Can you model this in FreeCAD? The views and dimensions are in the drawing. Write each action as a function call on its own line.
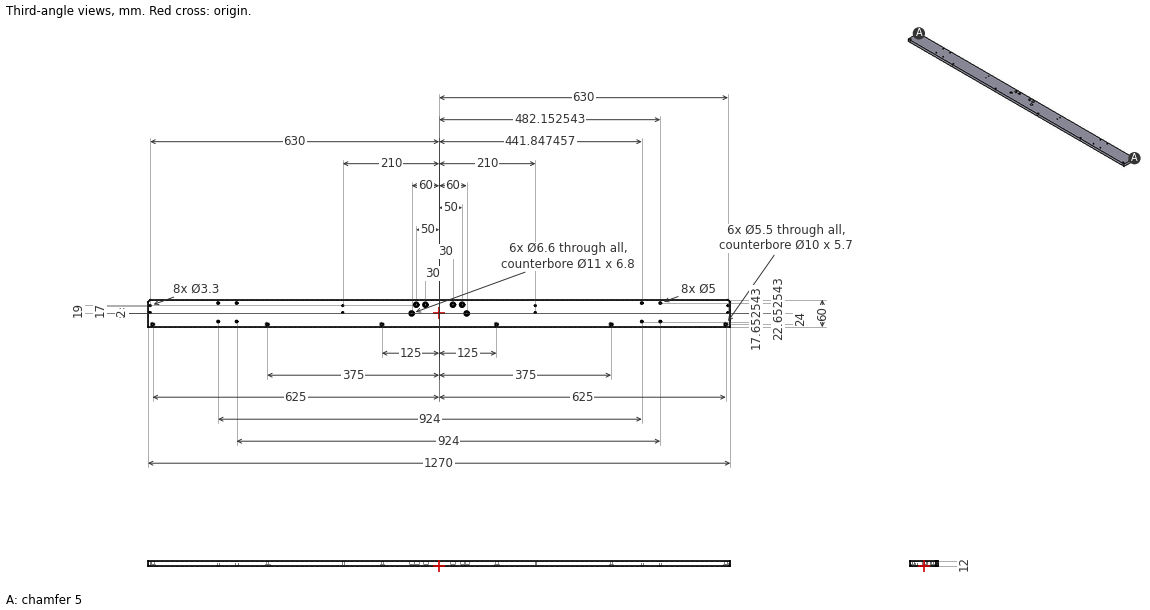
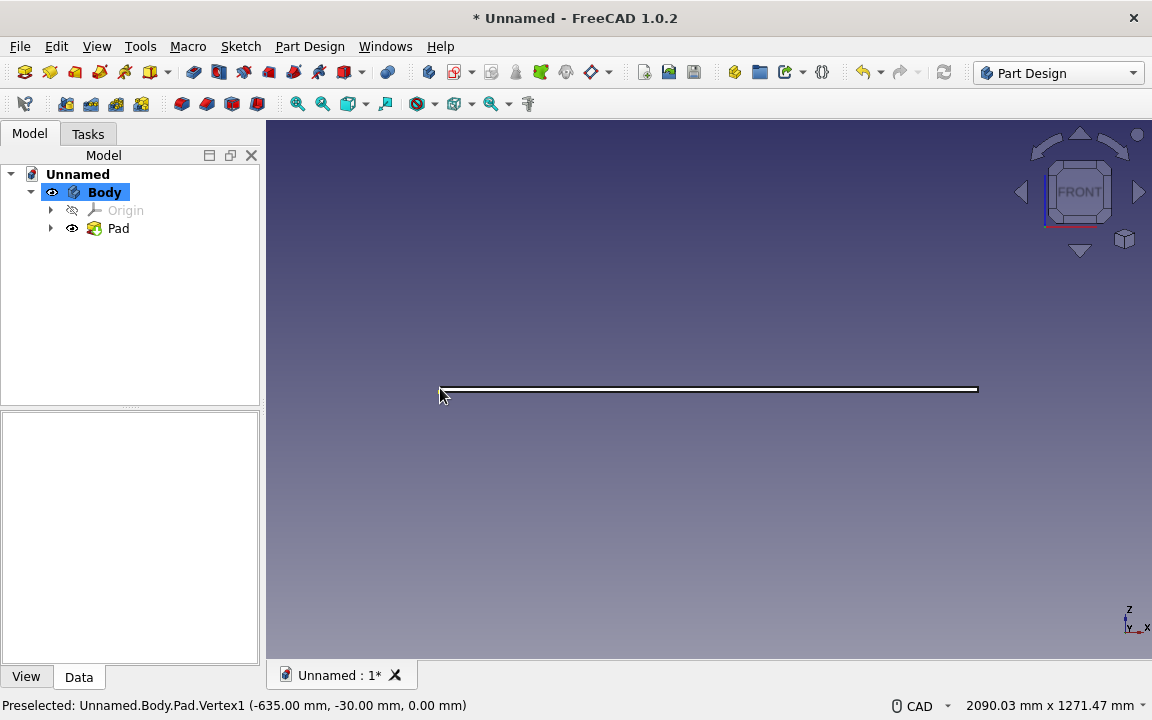
key(3)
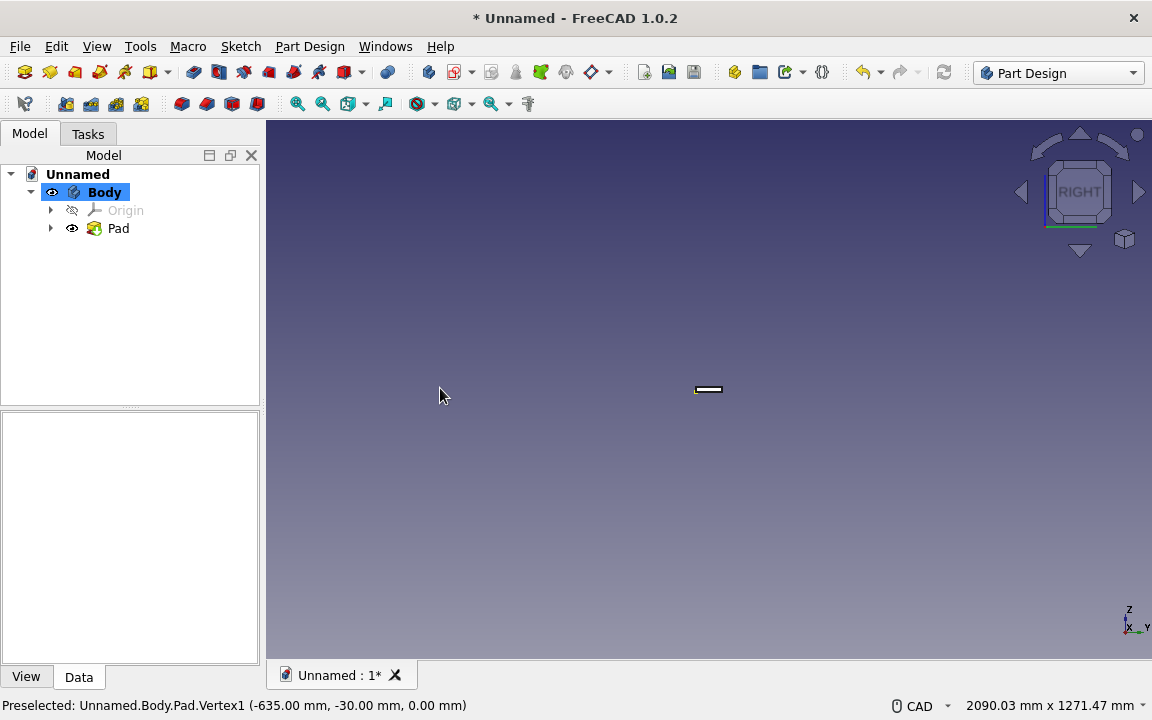
key(v)
key(f)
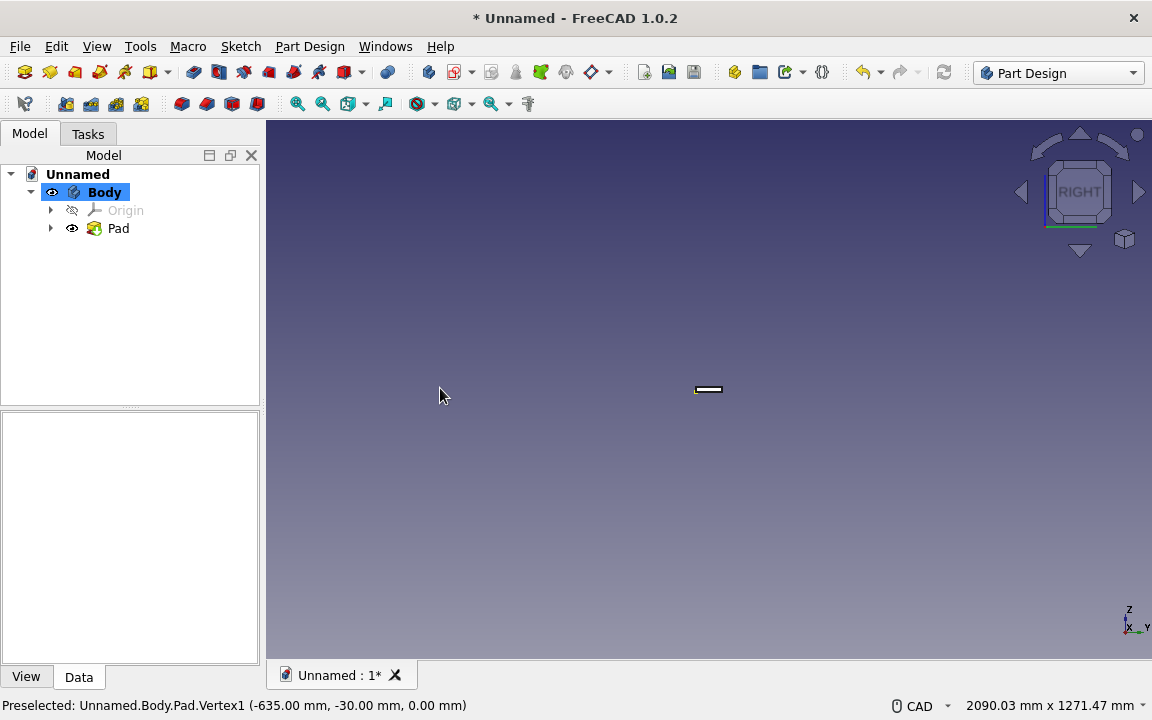
scroll(722, 388, up, 11)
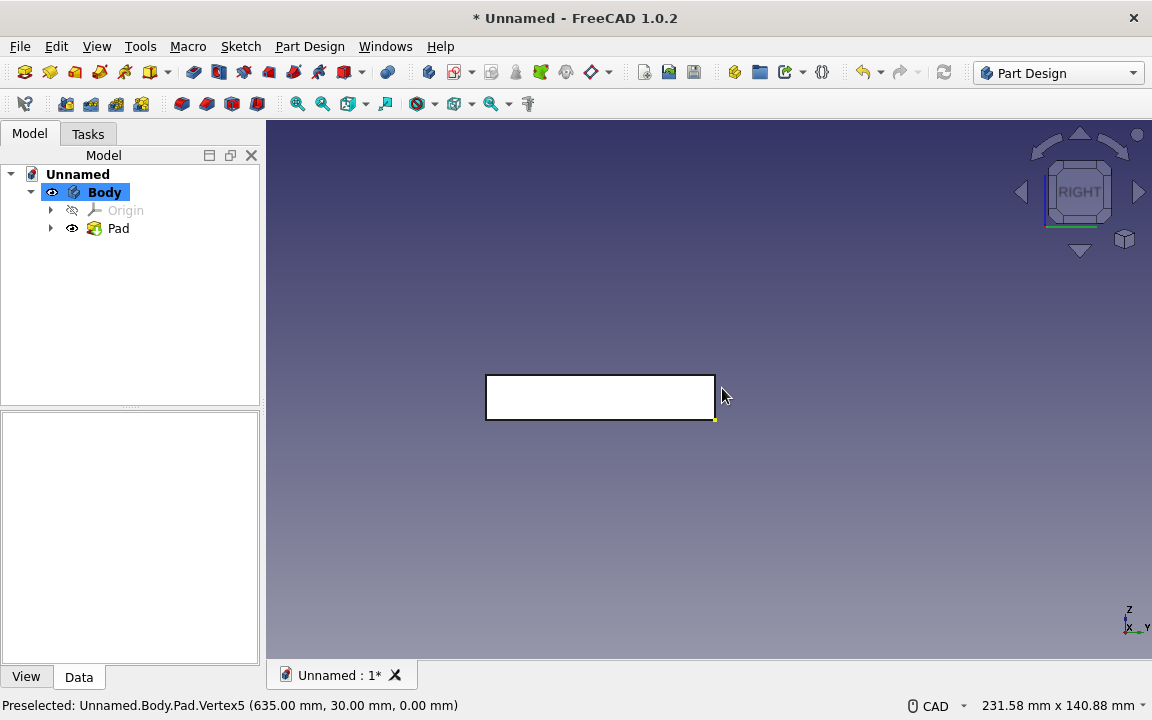
click(715, 397)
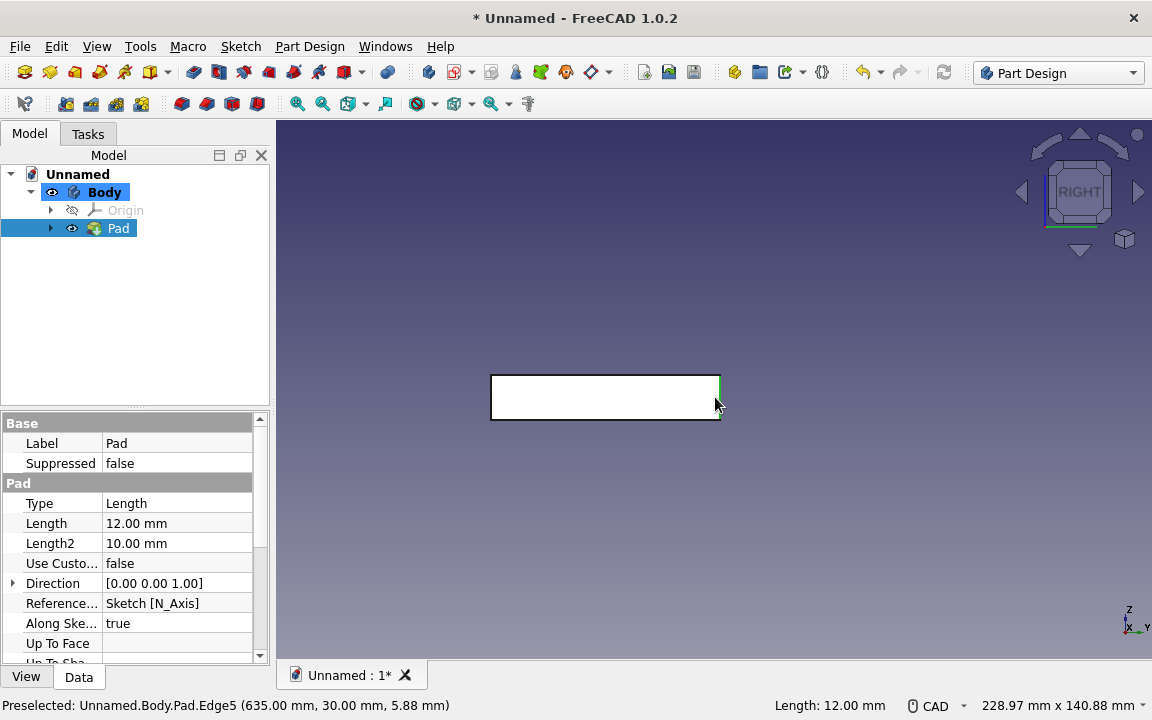
click(298, 104)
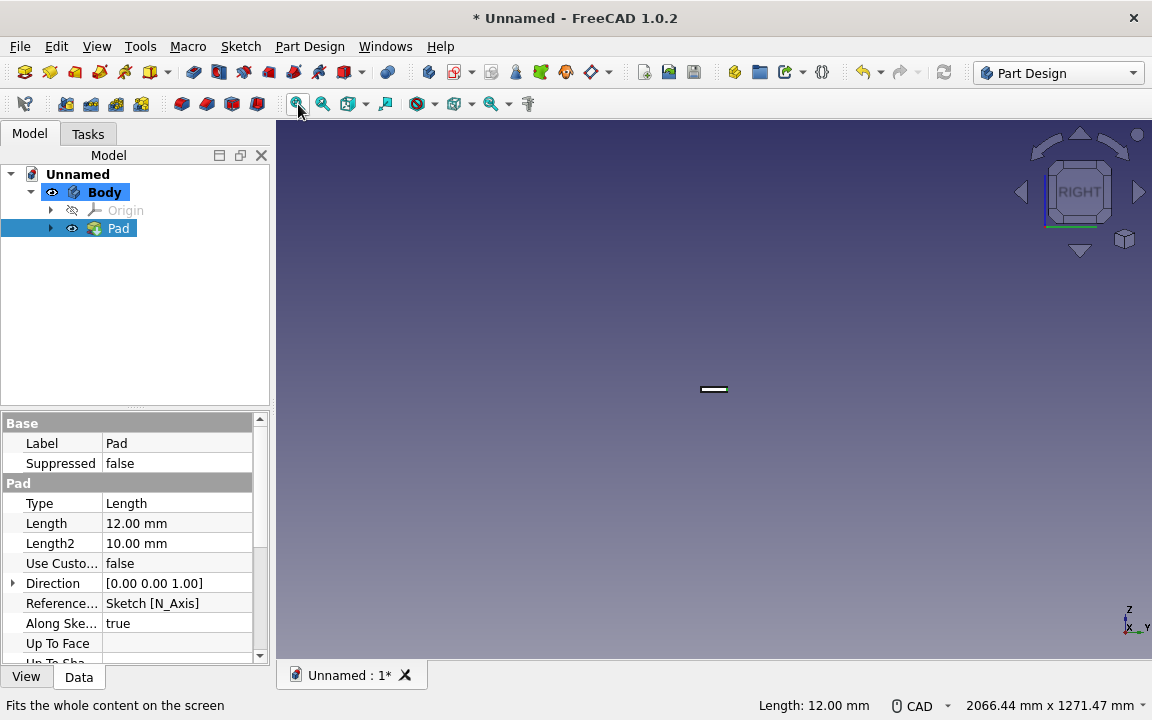
key(5)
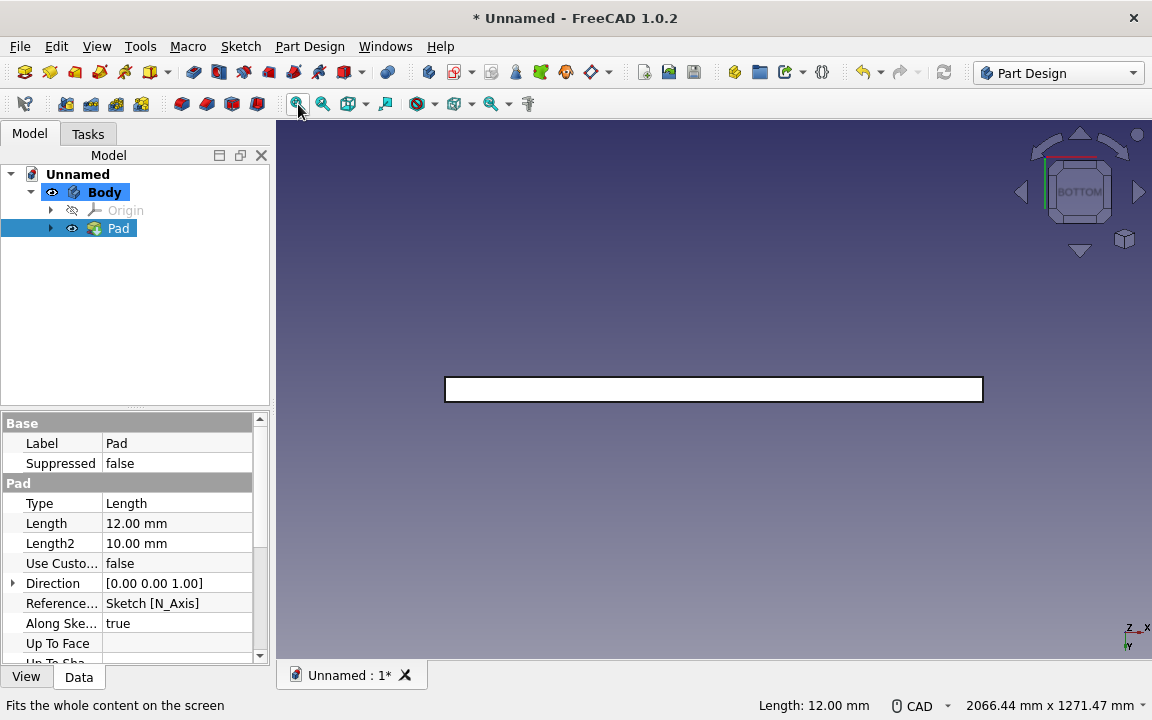
scroll(445, 401, up, 11)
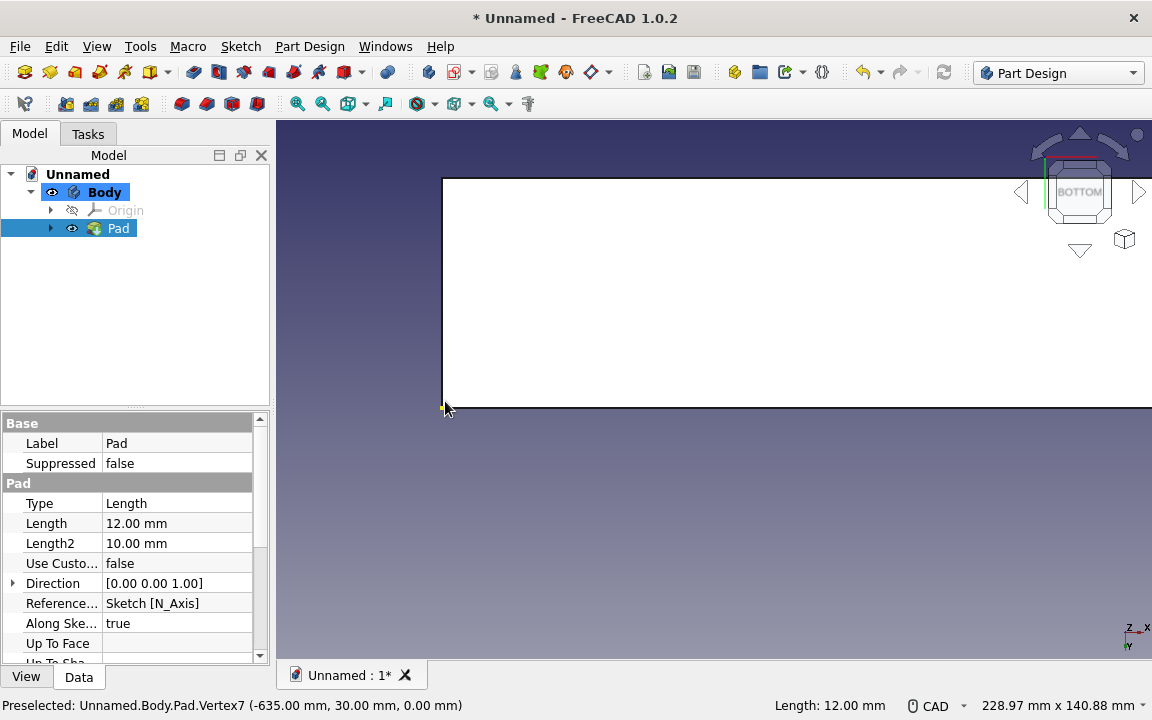
click(298, 104)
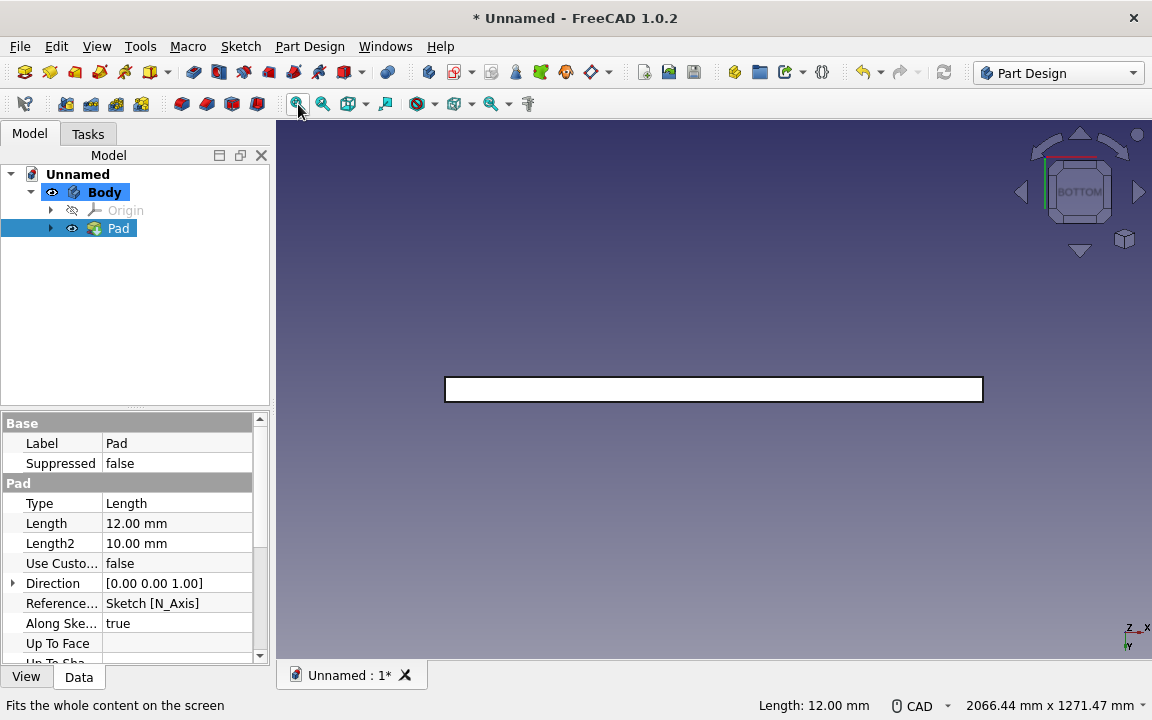
key(4)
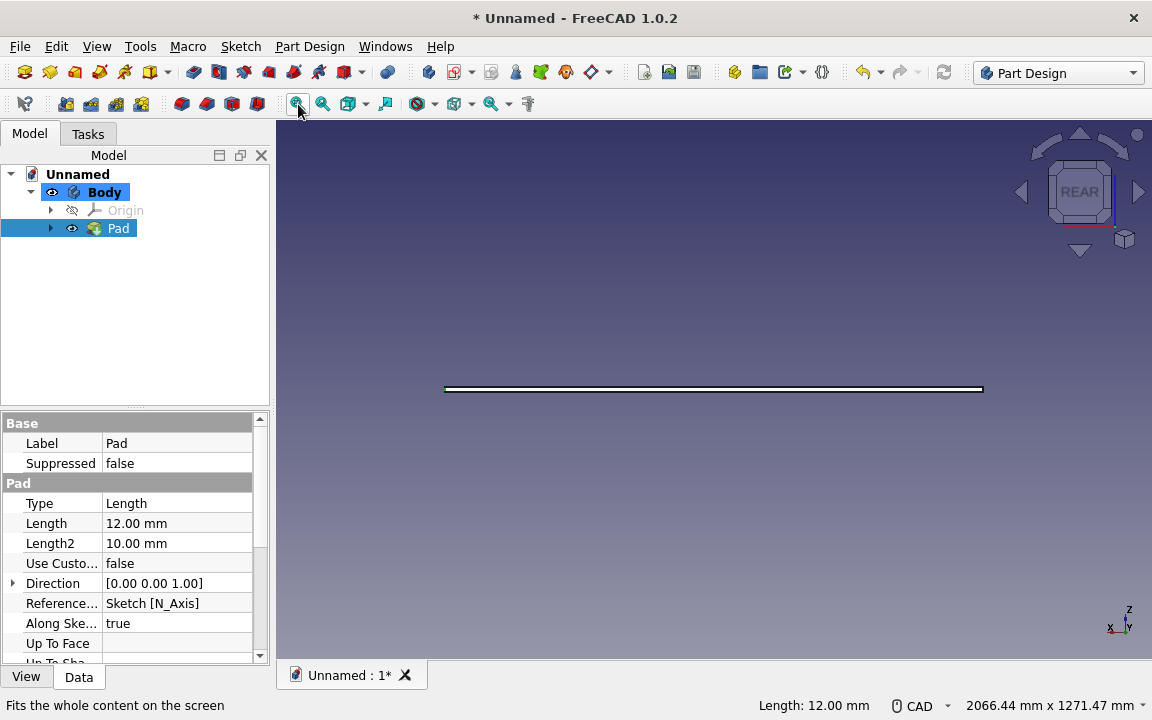
scroll(983, 388, up, 11)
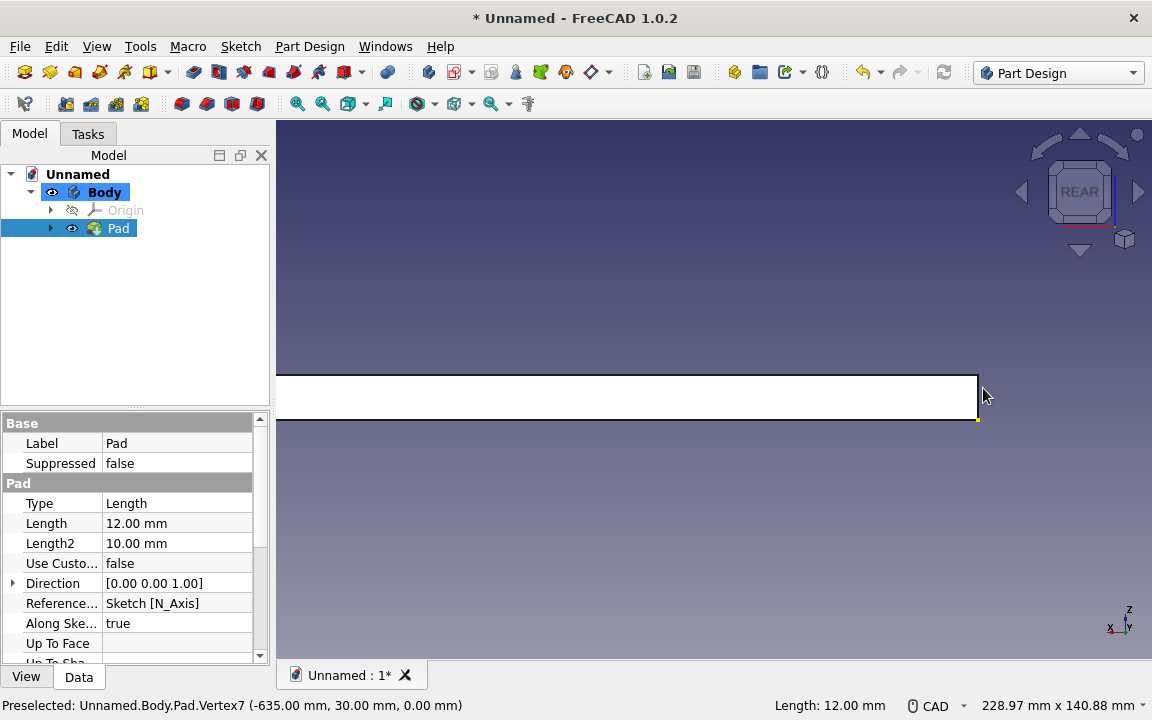
click(978, 397, ctrl)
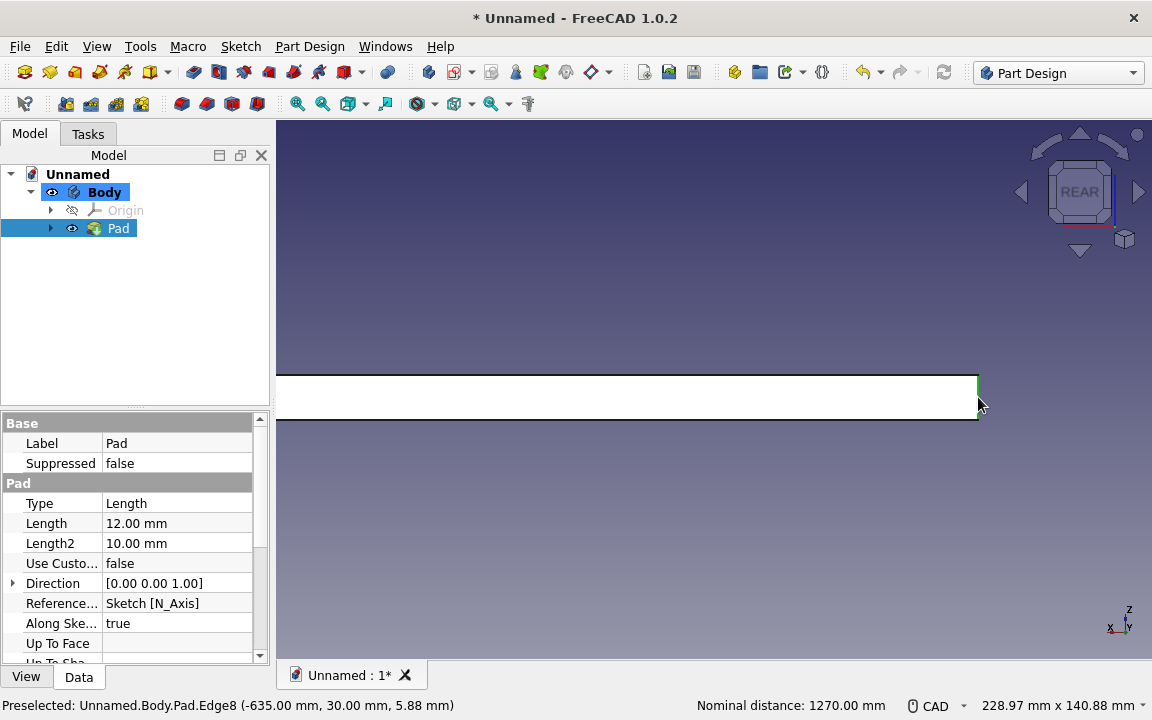
click(207, 104)